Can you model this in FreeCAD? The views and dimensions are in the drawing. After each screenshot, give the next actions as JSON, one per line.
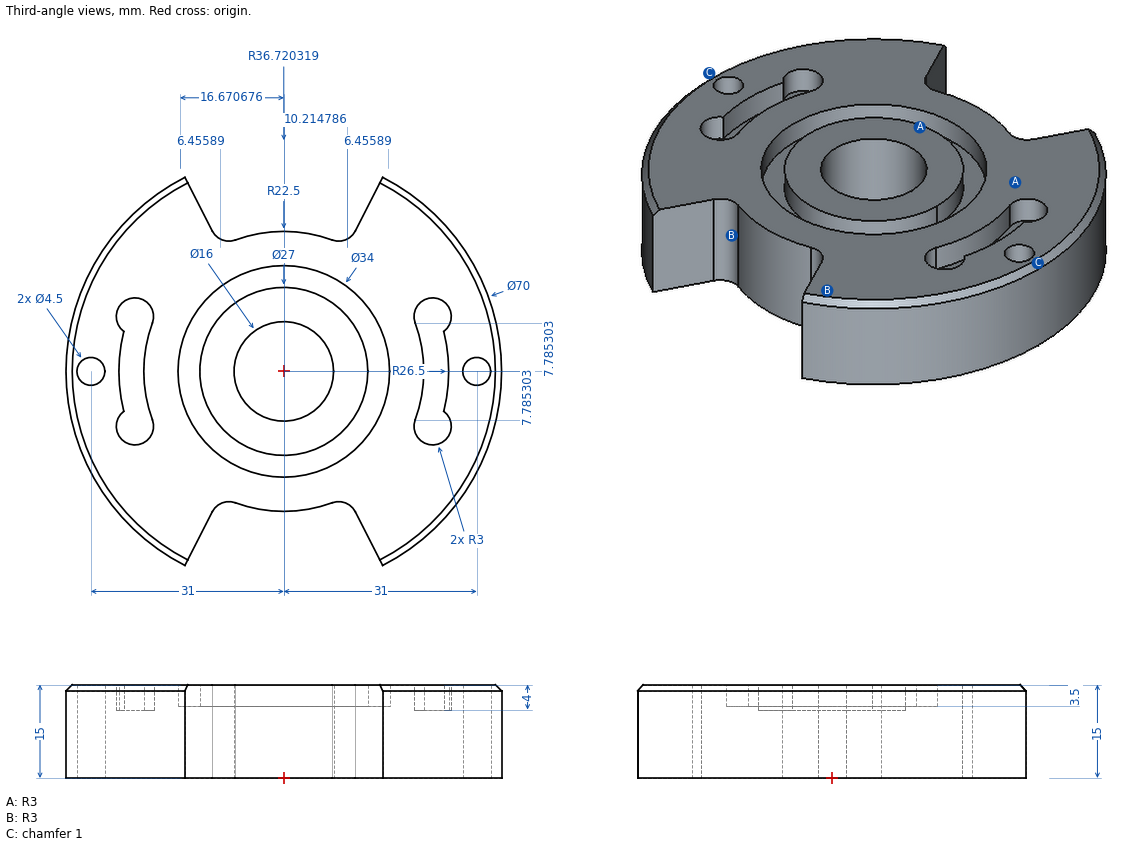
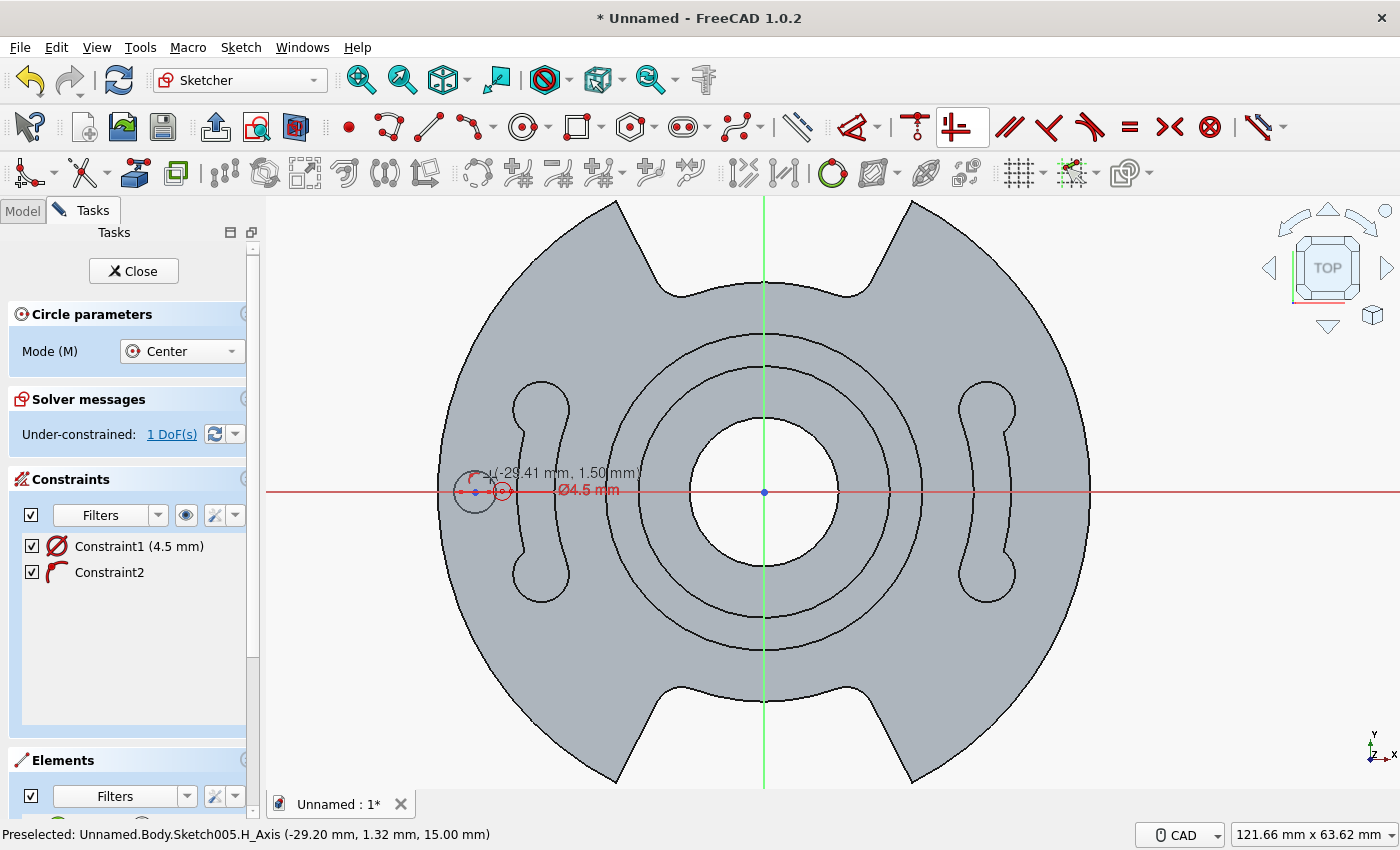
{"action": "left_click", "coordinate": [1053, 492]}
{"action": "mouse_move", "coordinate": [1068, 477]}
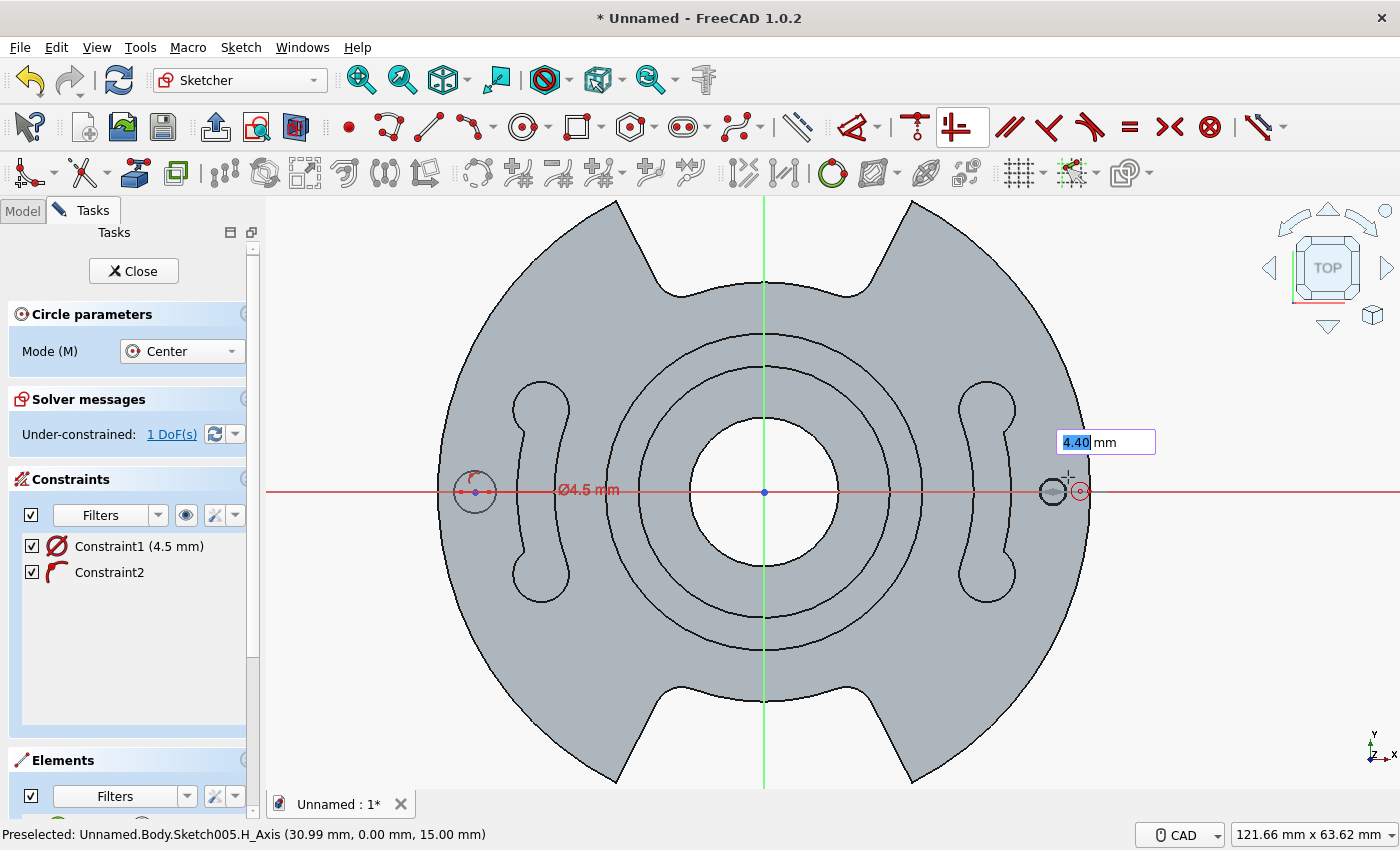
{"action": "type", "text": "4.5"}
{"action": "key", "text": "Return"}
{"action": "key", "text": "Escape"}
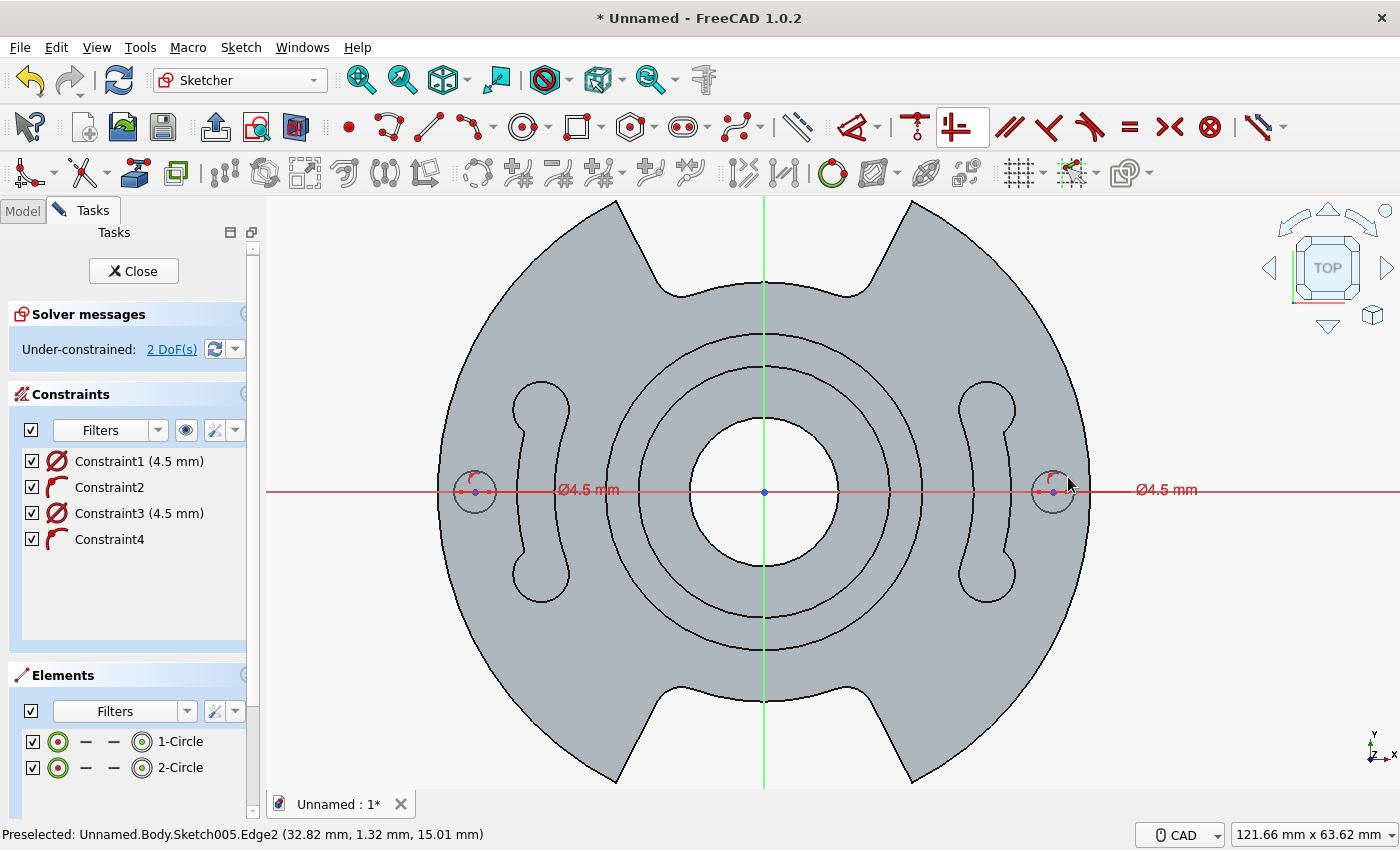
{"action": "key", "text": "d"}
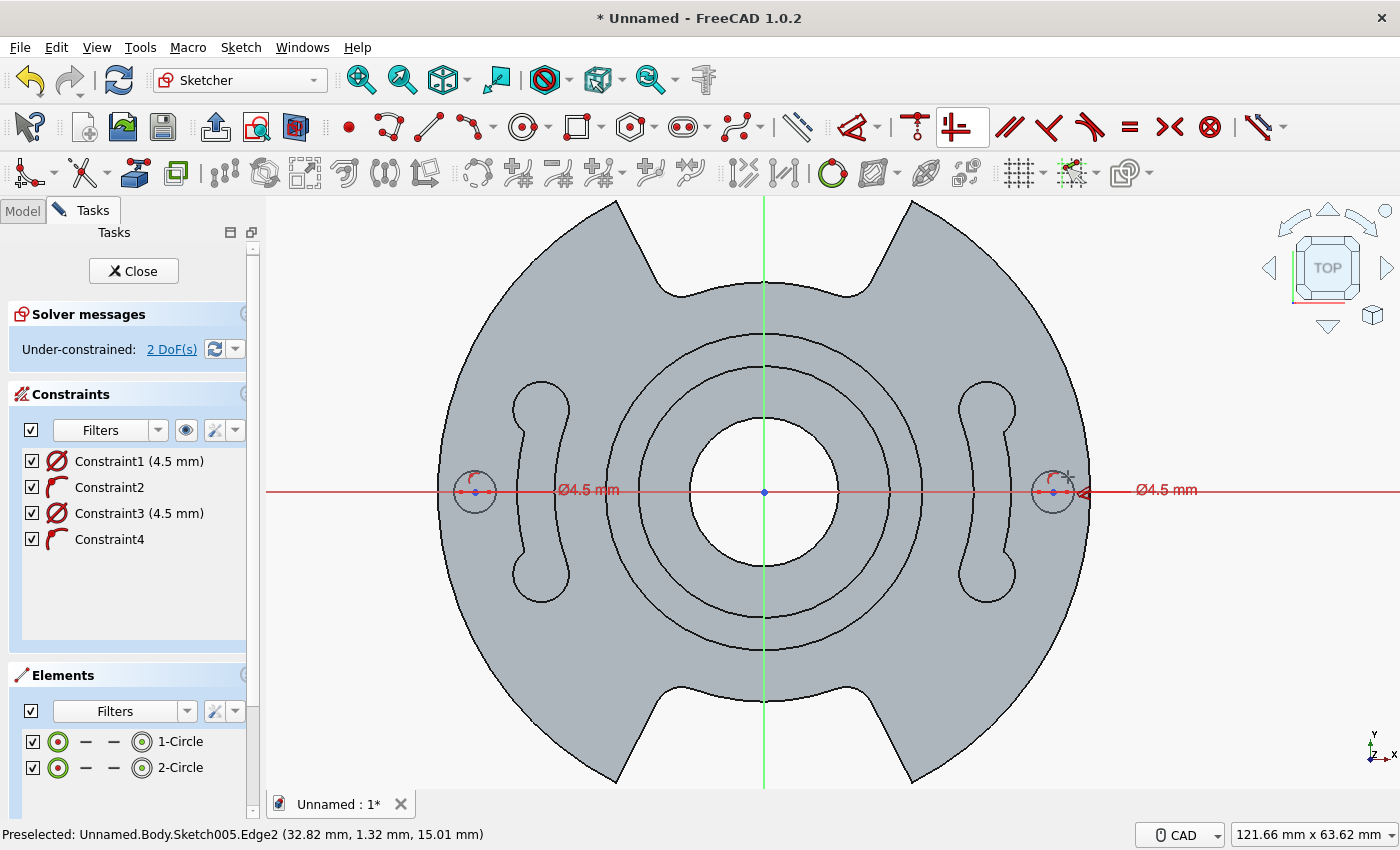
{"action": "left_click", "coordinate": [475, 492]}
{"action": "left_click", "coordinate": [620, 526]}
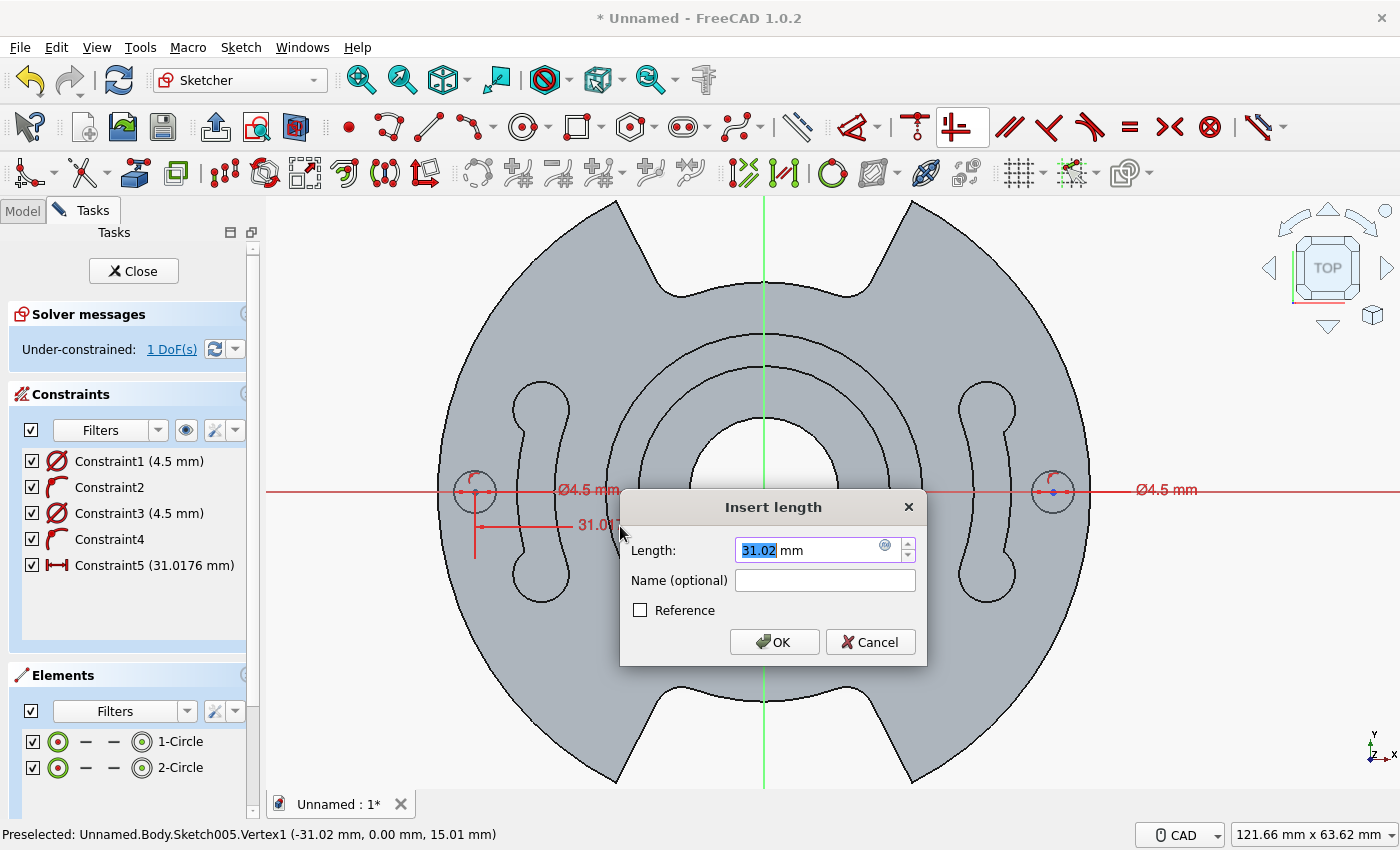
{"action": "type", "text": "31"}
{"action": "key", "text": "Return"}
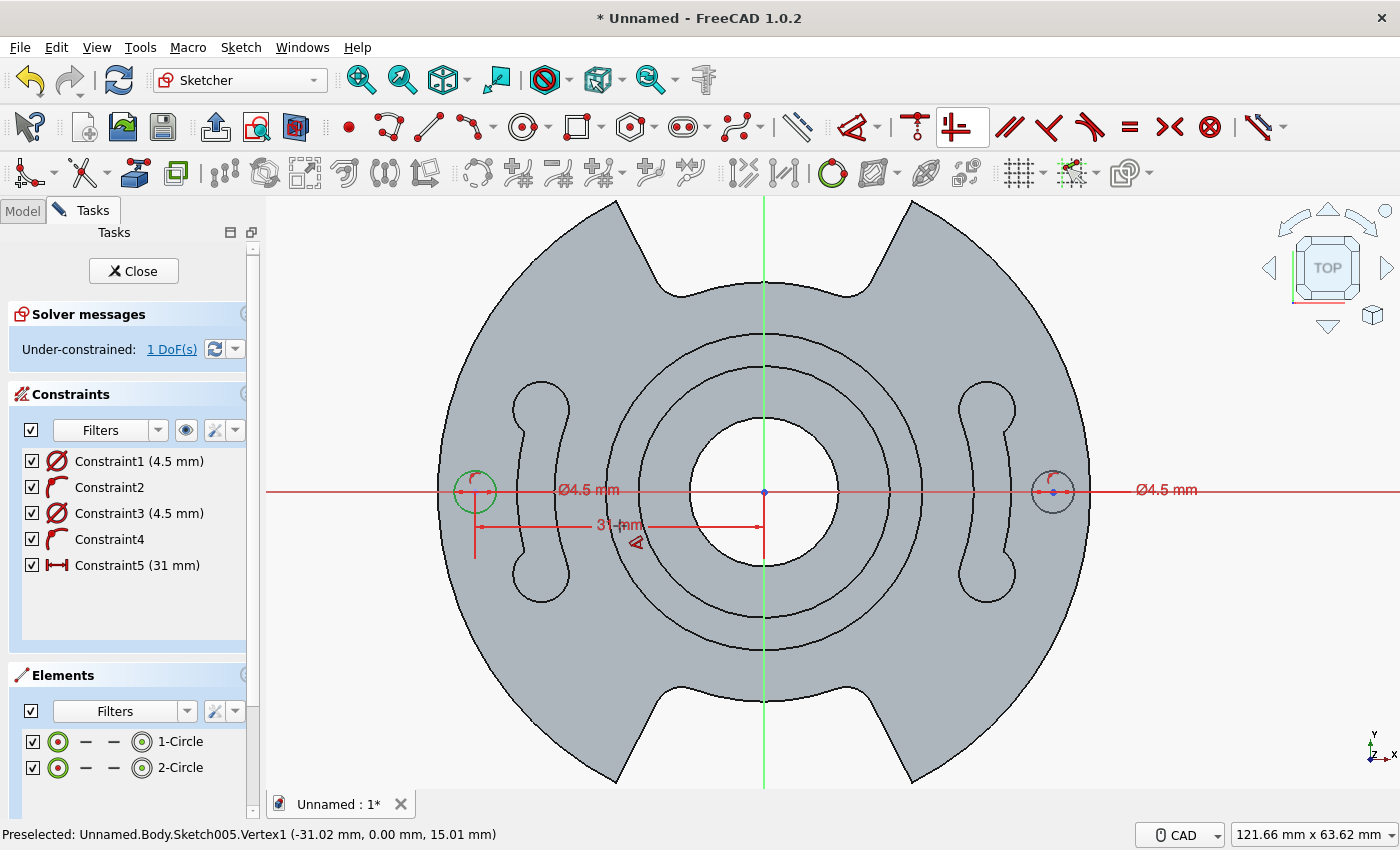
{"action": "left_click", "coordinate": [1053, 492]}
{"action": "left_click", "coordinate": [909, 526]}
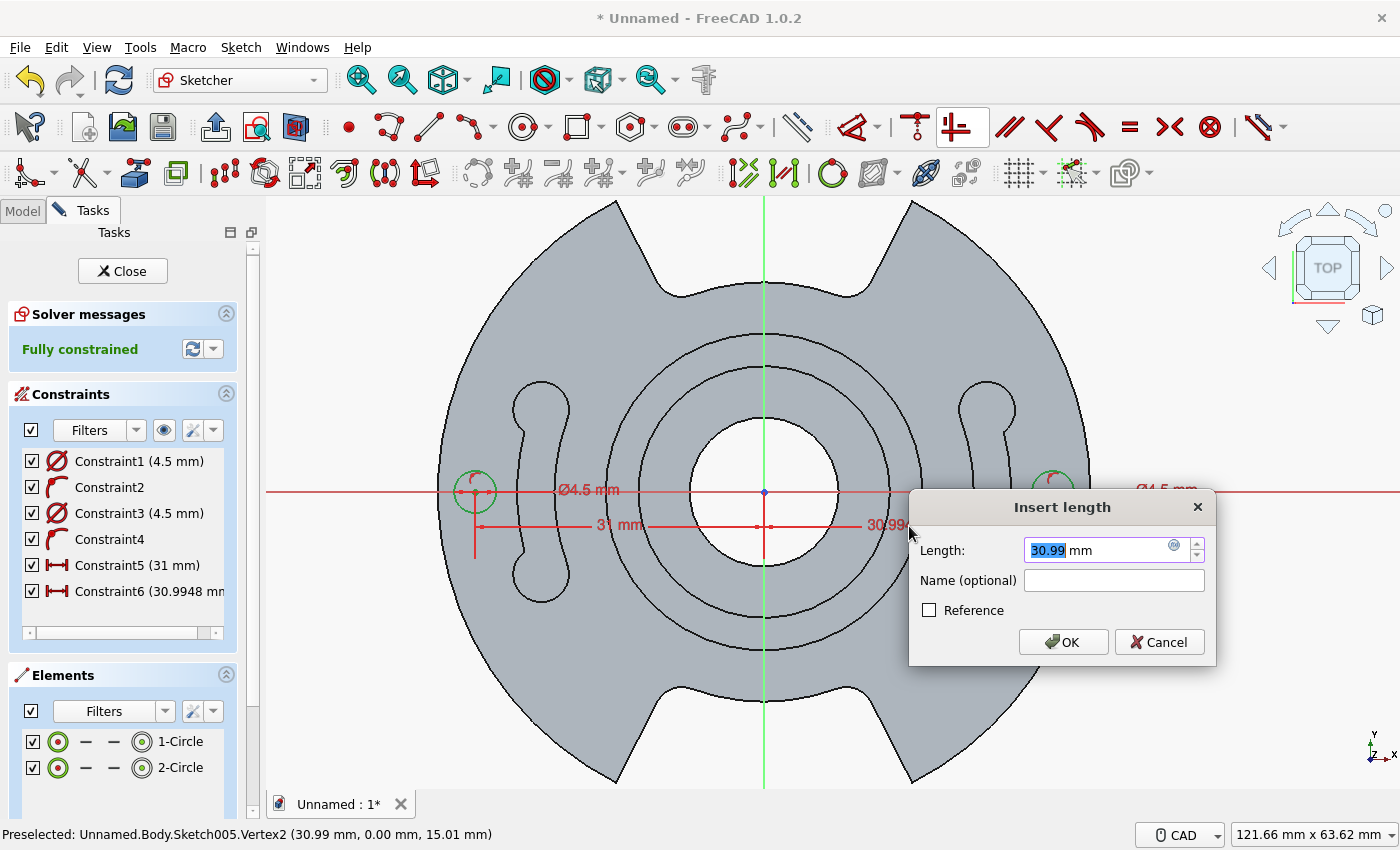
{"action": "type", "text": "31"}
{"action": "key", "text": "Return"}
{"action": "key", "text": "Escape"}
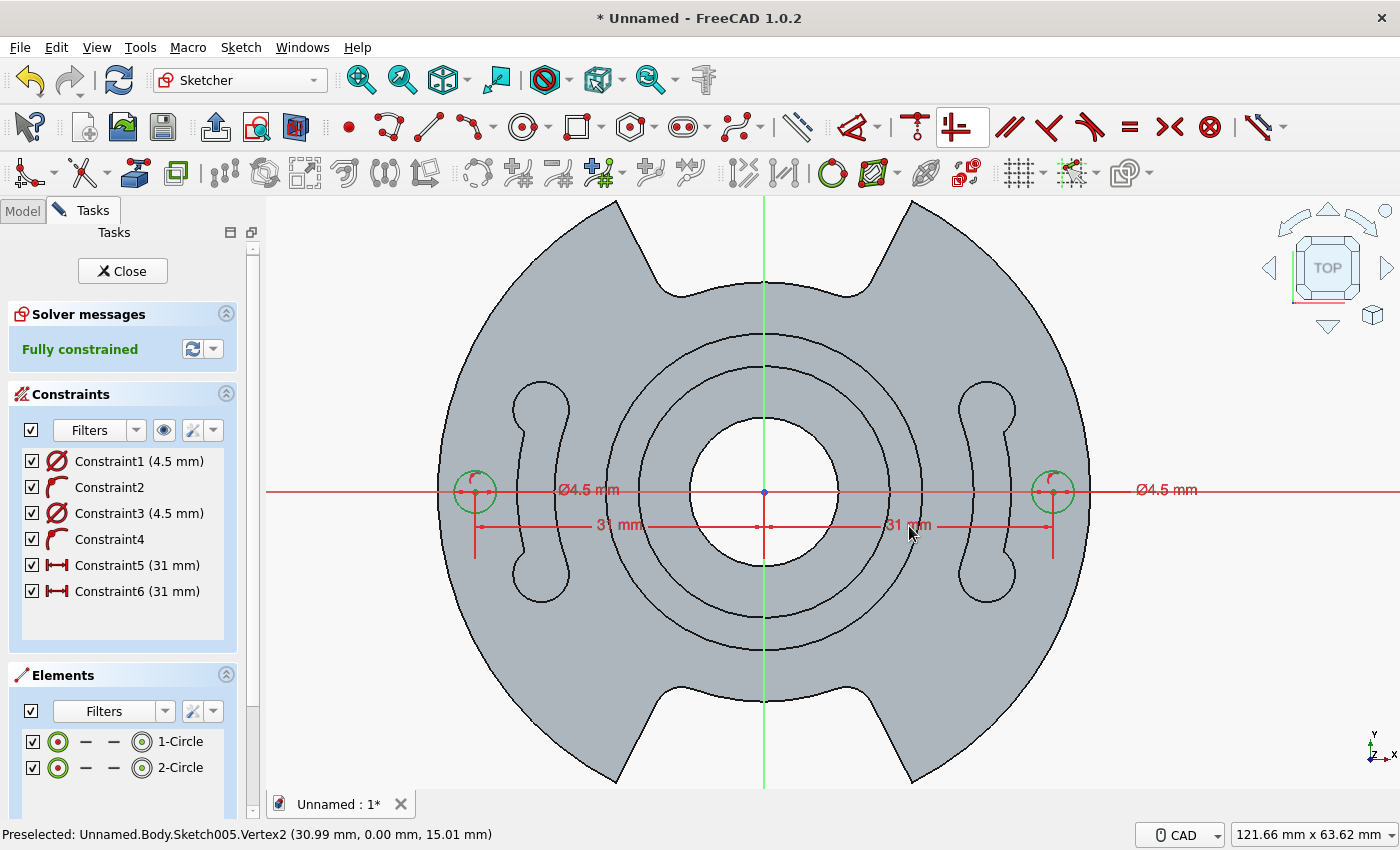
{"action": "left_click", "coordinate": [123, 271]}